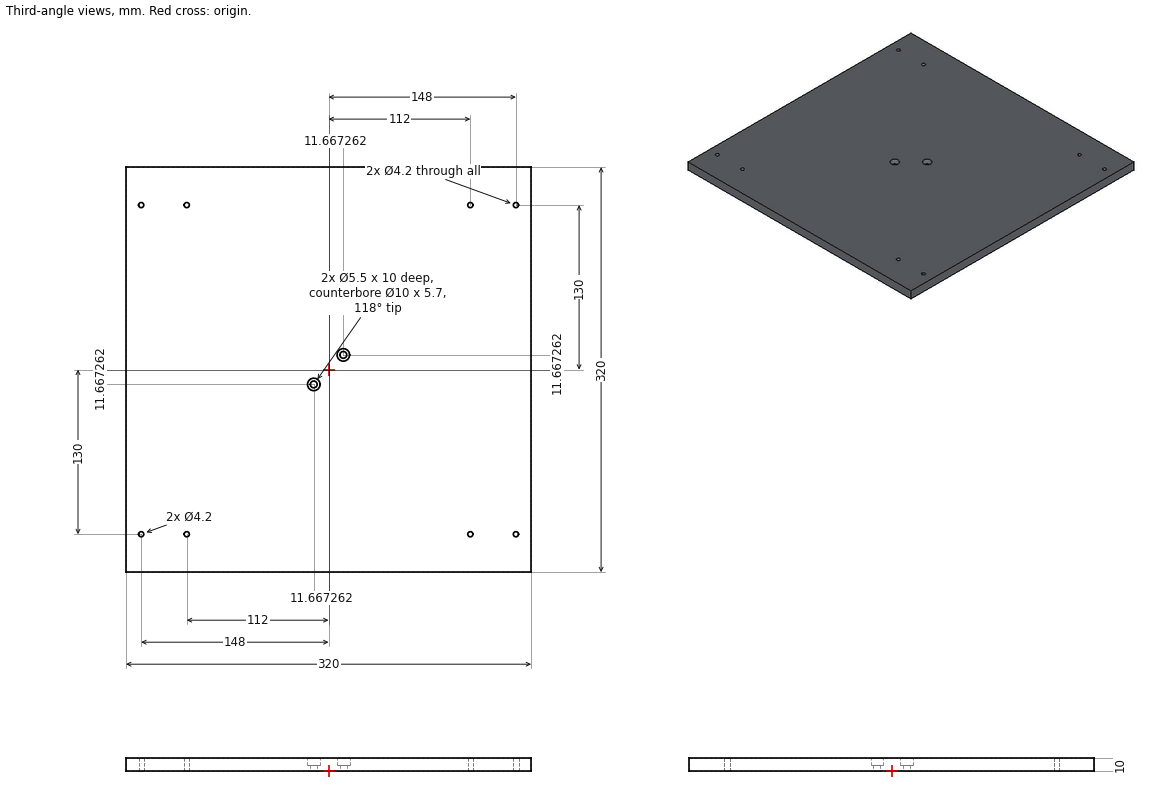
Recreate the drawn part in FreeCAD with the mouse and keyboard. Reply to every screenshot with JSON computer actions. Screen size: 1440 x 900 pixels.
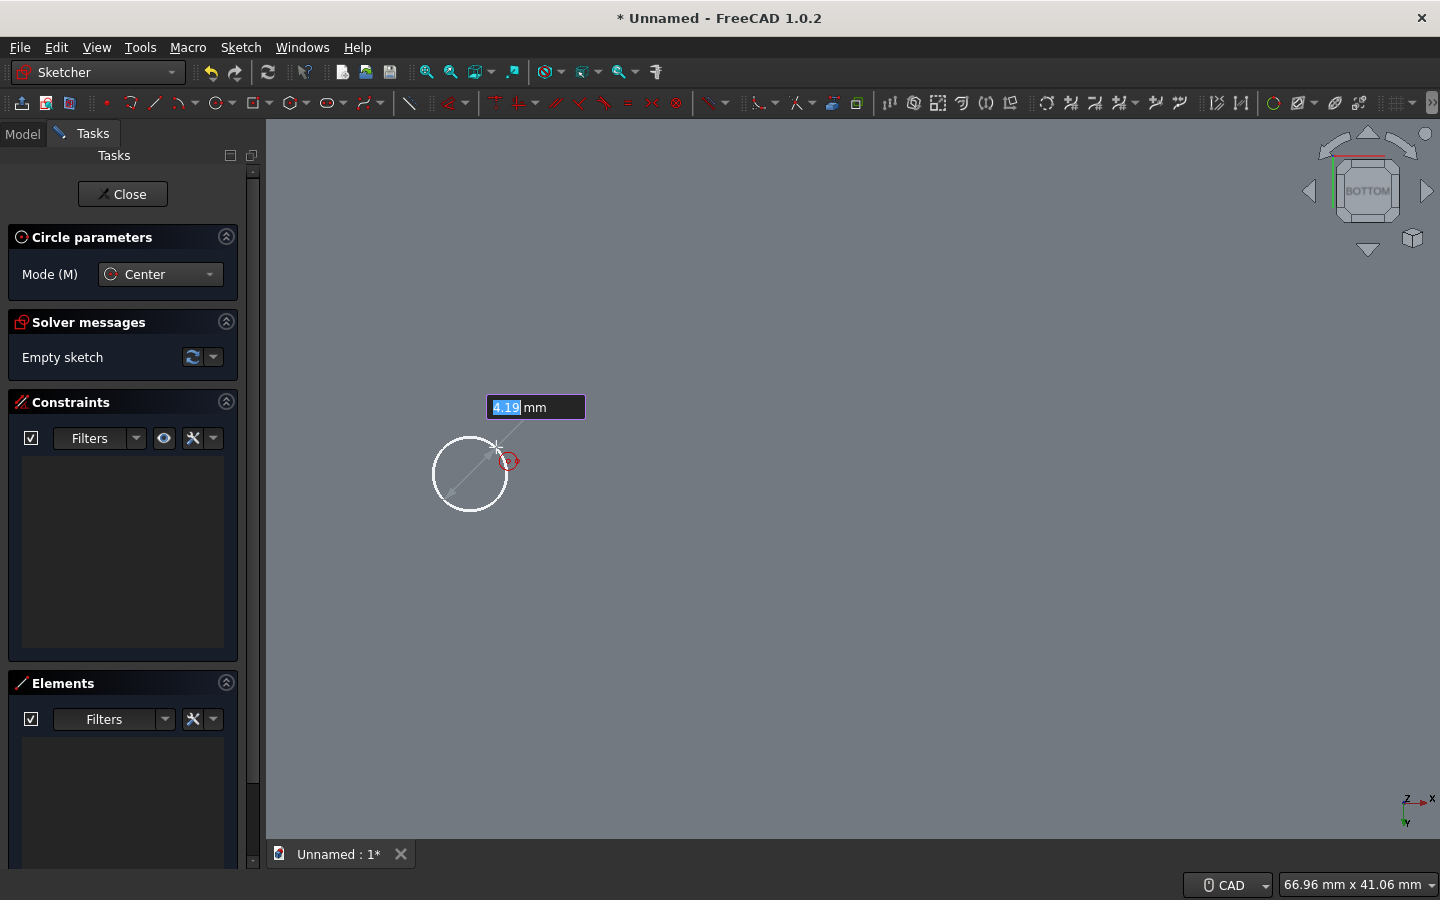
{"action": "type", "text": "4.2"}
{"action": "key", "text": "Return"}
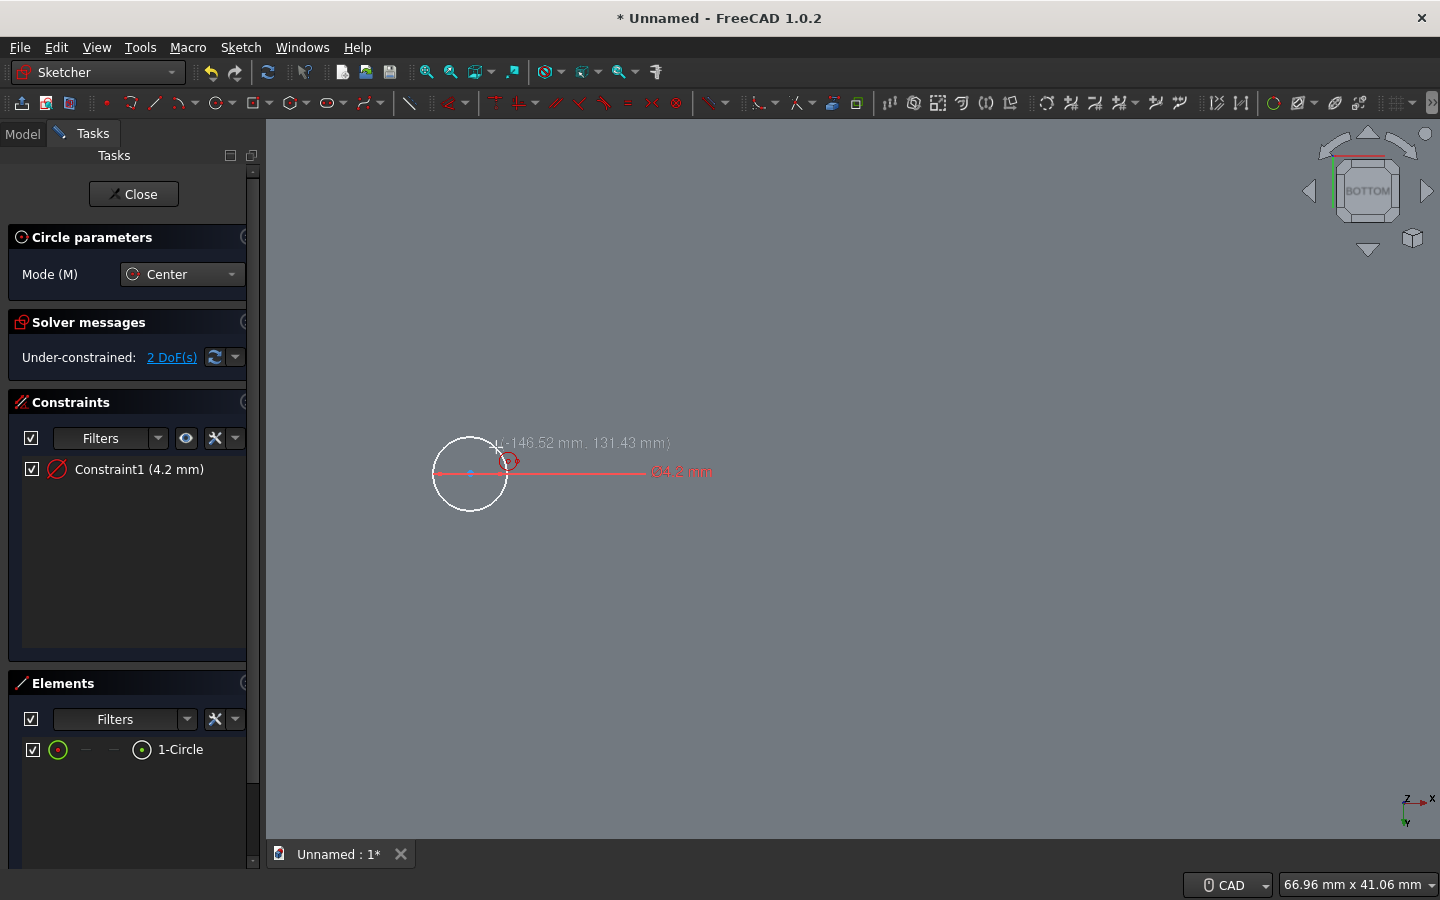
{"action": "left_click", "coordinate": [1101, 473]}
{"action": "mouse_move", "coordinate": [1127, 447]}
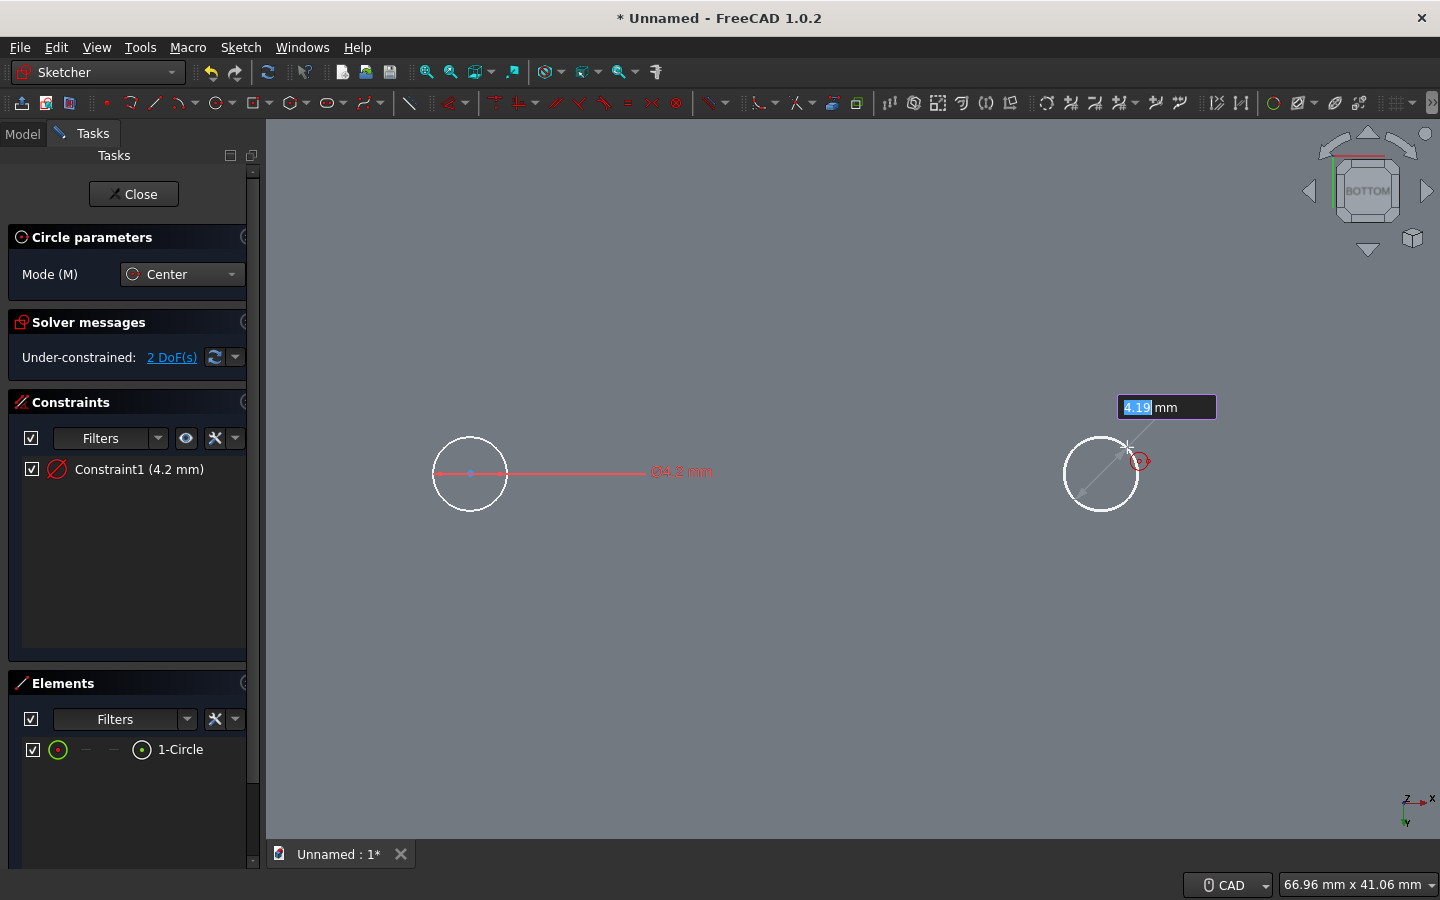
{"action": "type", "text": "4.2"}
{"action": "key", "text": "Return"}
{"action": "key", "text": "Escape"}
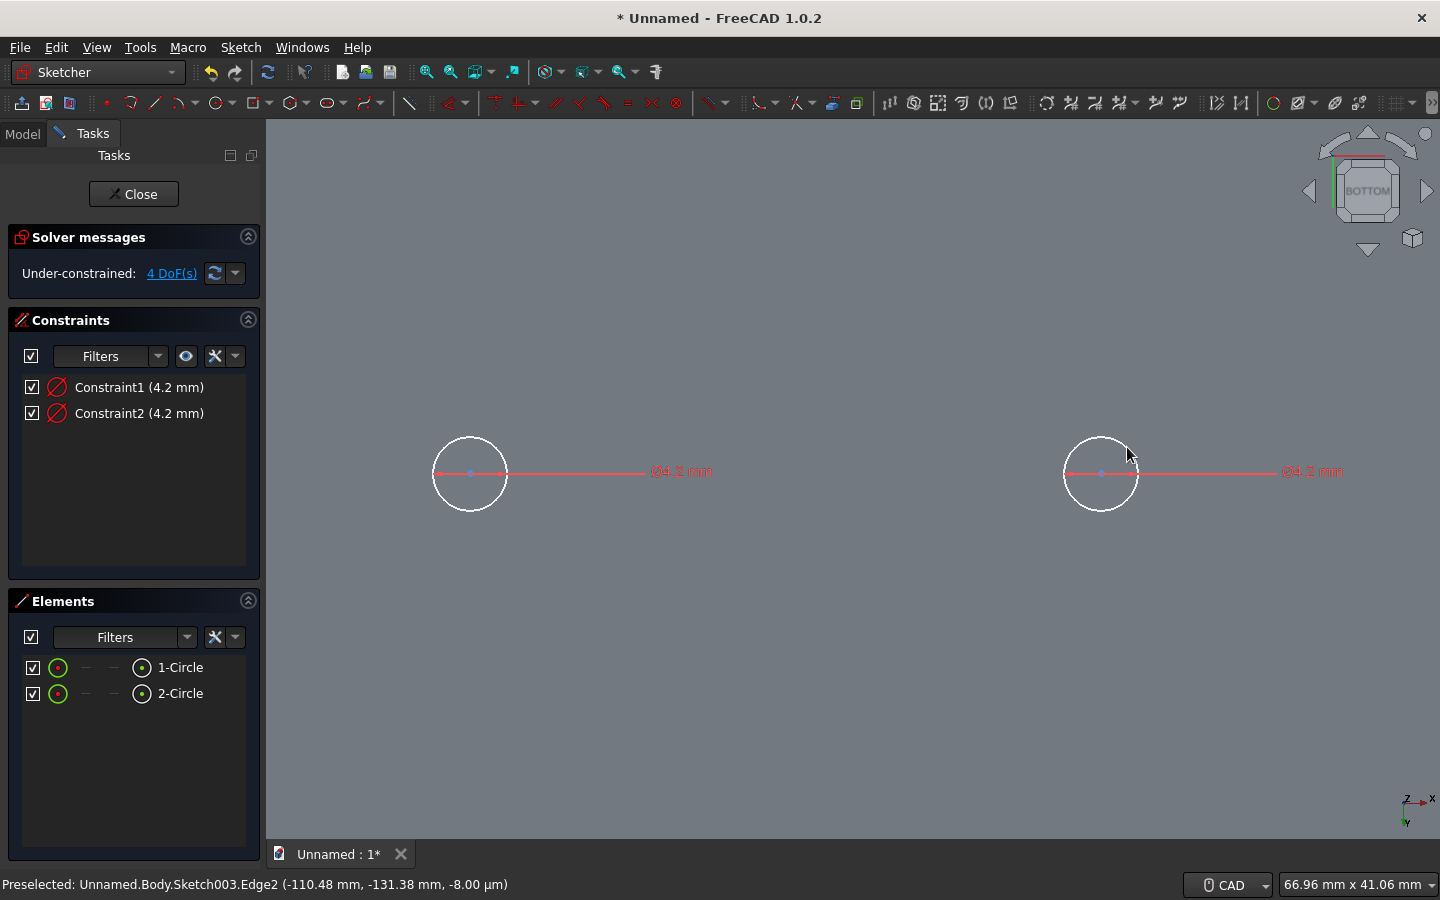
{"action": "key", "text": "d"}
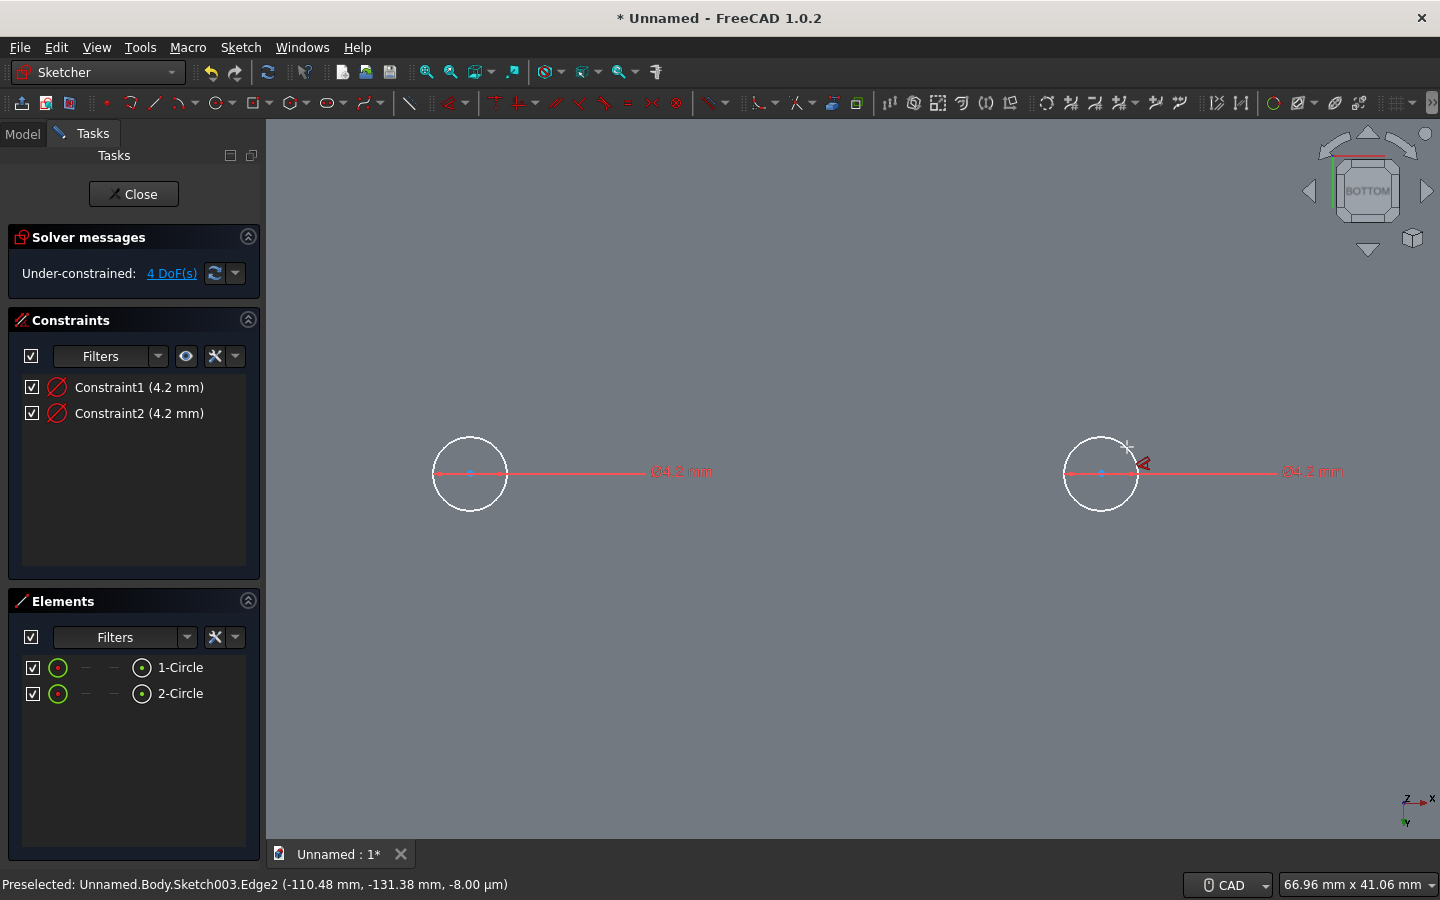
{"action": "left_click", "coordinate": [470, 474]}
{"action": "left_click", "coordinate": [873, 440]}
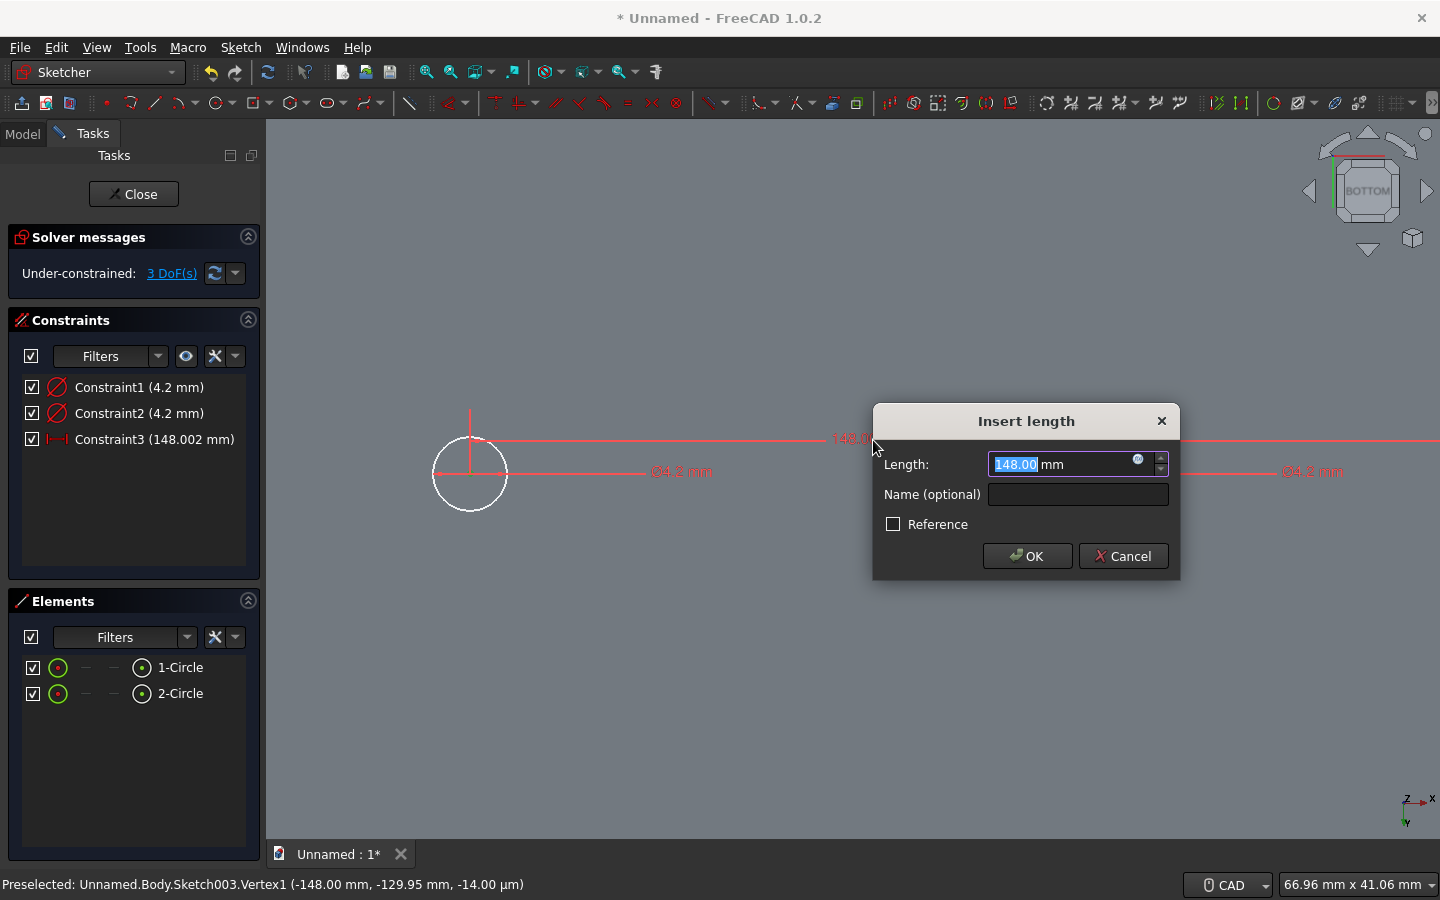
{"action": "type", "text": "148"}
{"action": "key", "text": "Return"}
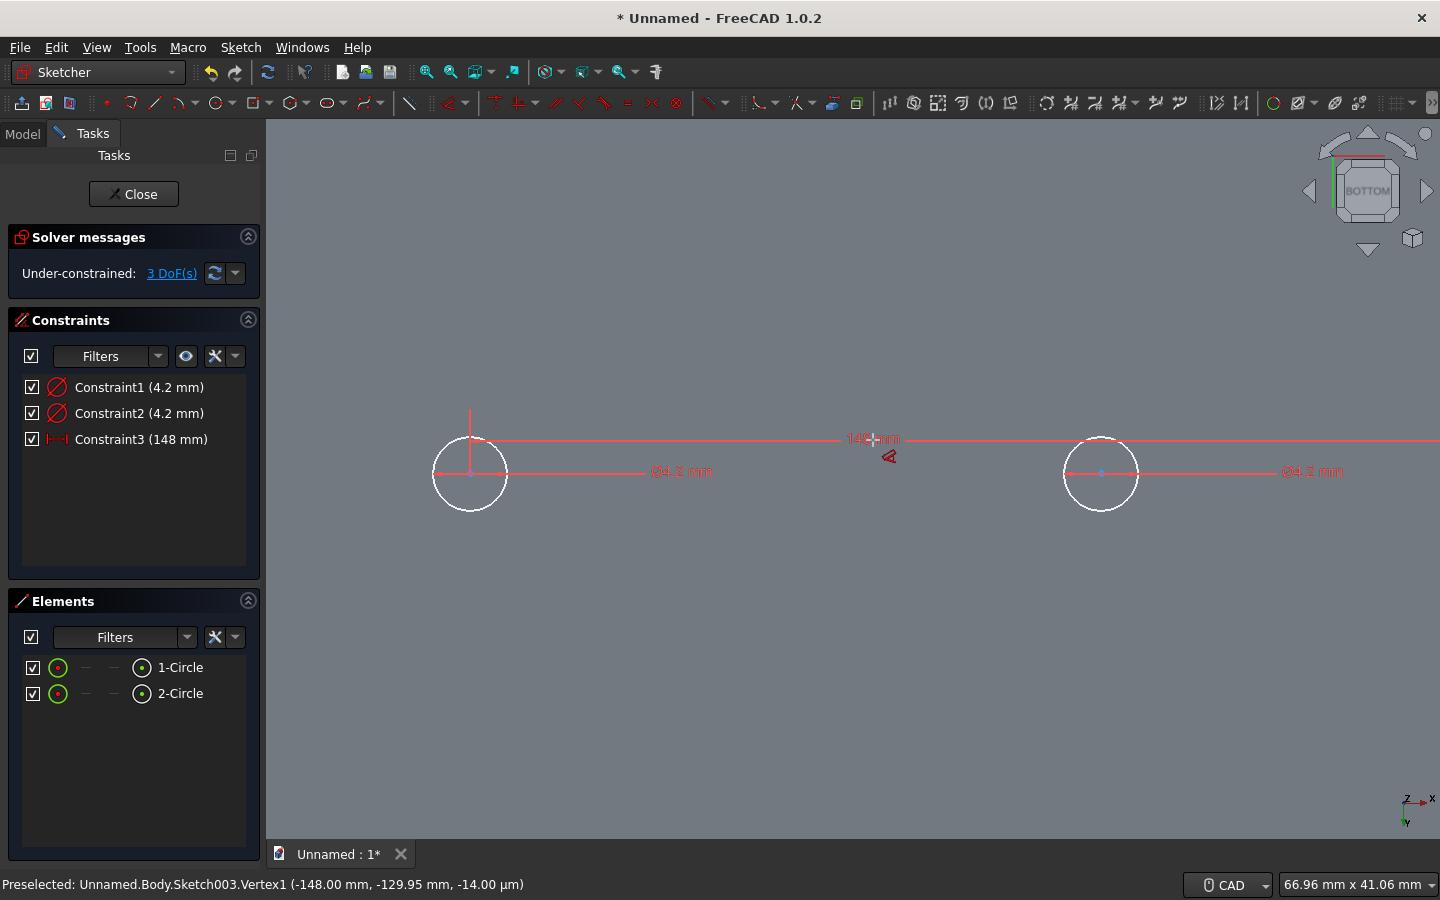
{"action": "left_click", "coordinate": [470, 474]}
{"action": "left_click", "coordinate": [436, 642]}